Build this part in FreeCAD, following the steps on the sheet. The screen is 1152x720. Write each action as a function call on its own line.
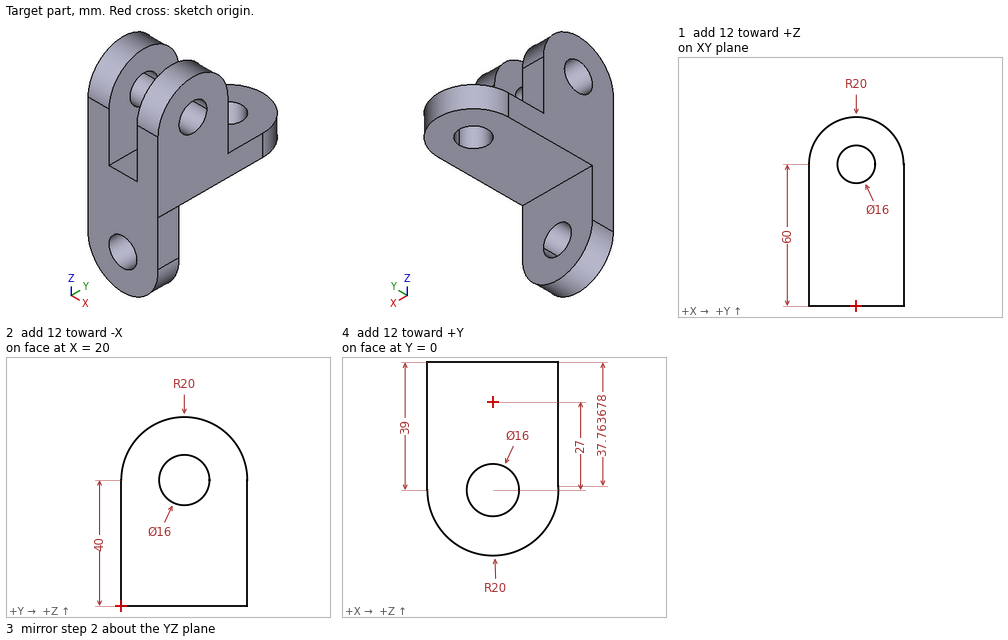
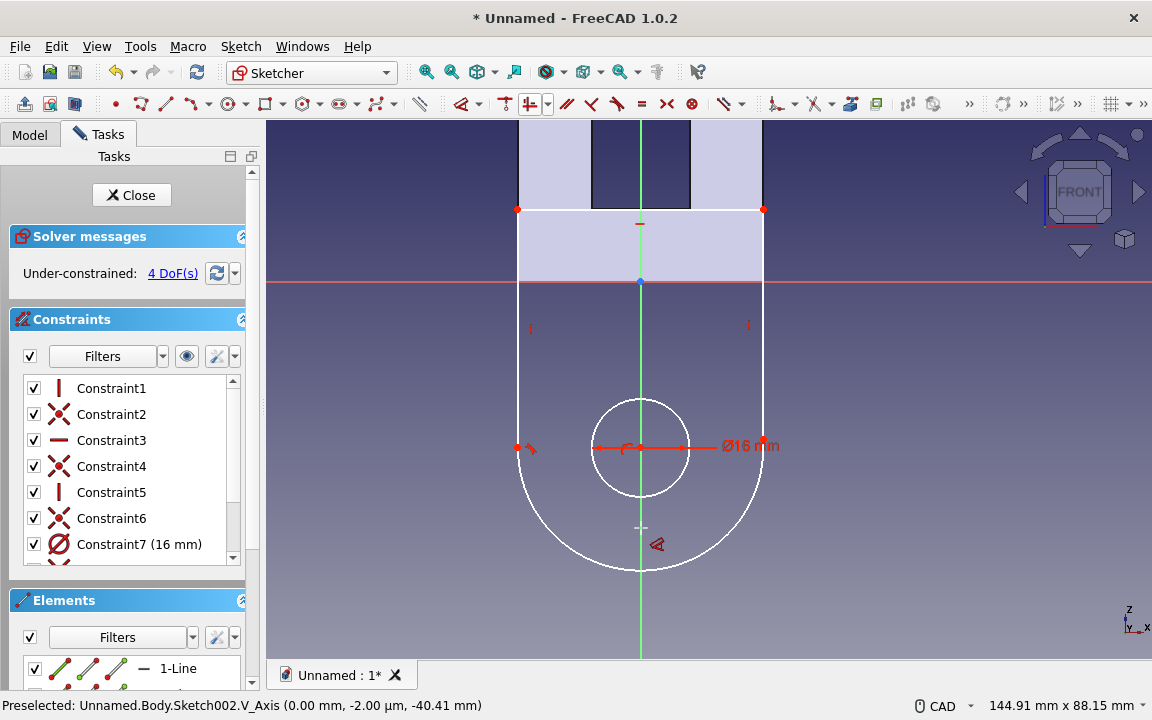
click(570, 549)
click(552, 575)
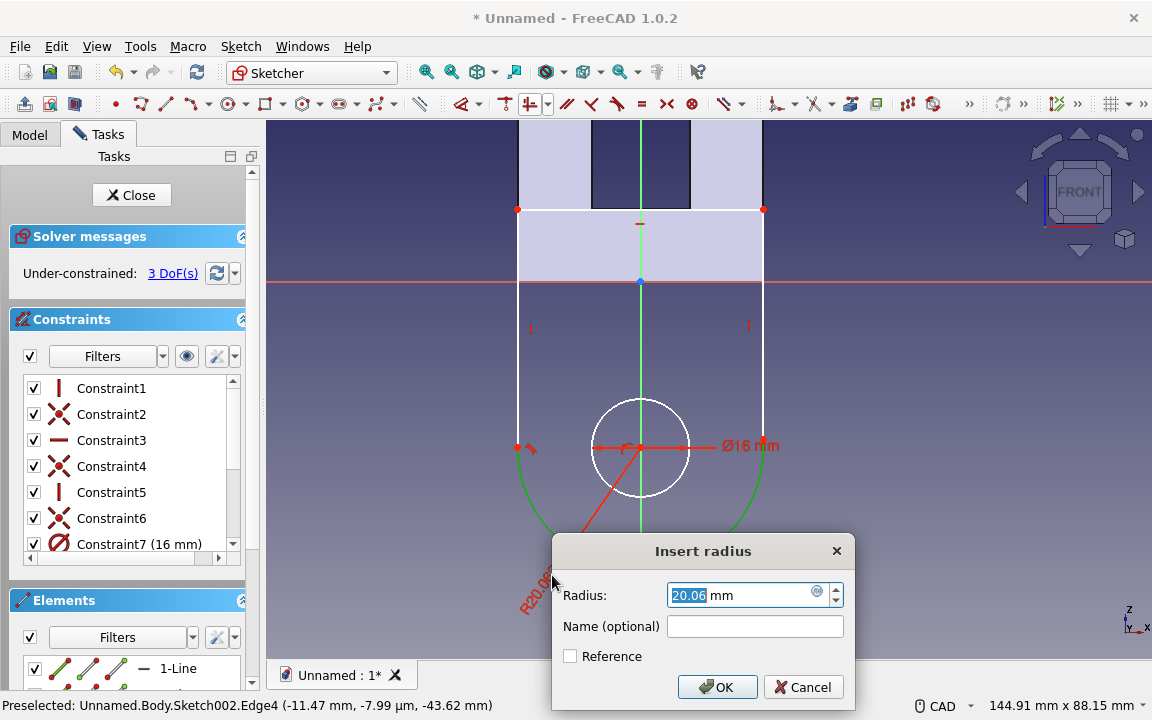
text(20)
key(Return)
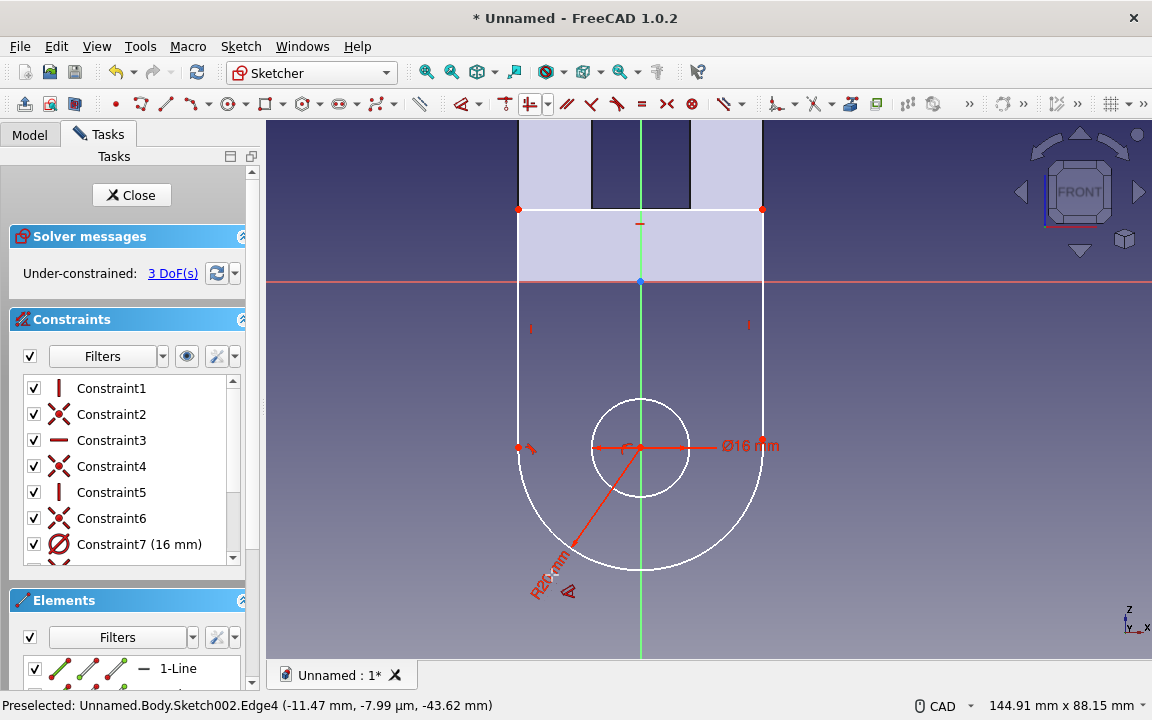
click(518, 281)
click(484, 329)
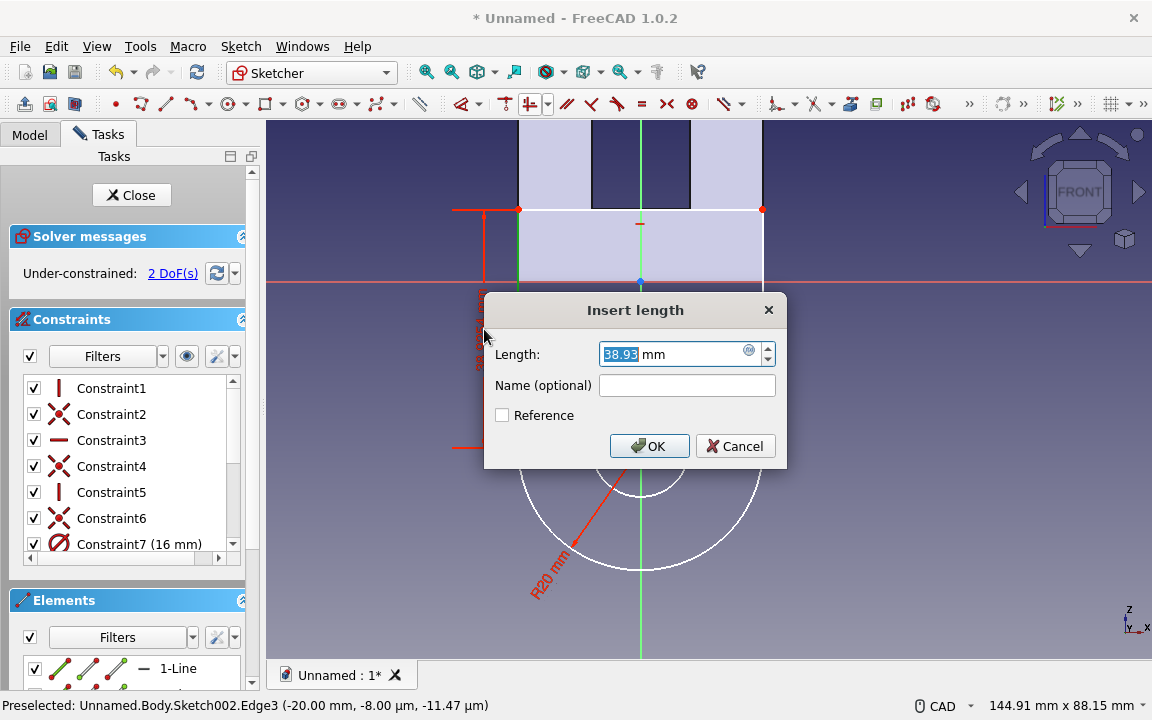
text(39)
key(Return)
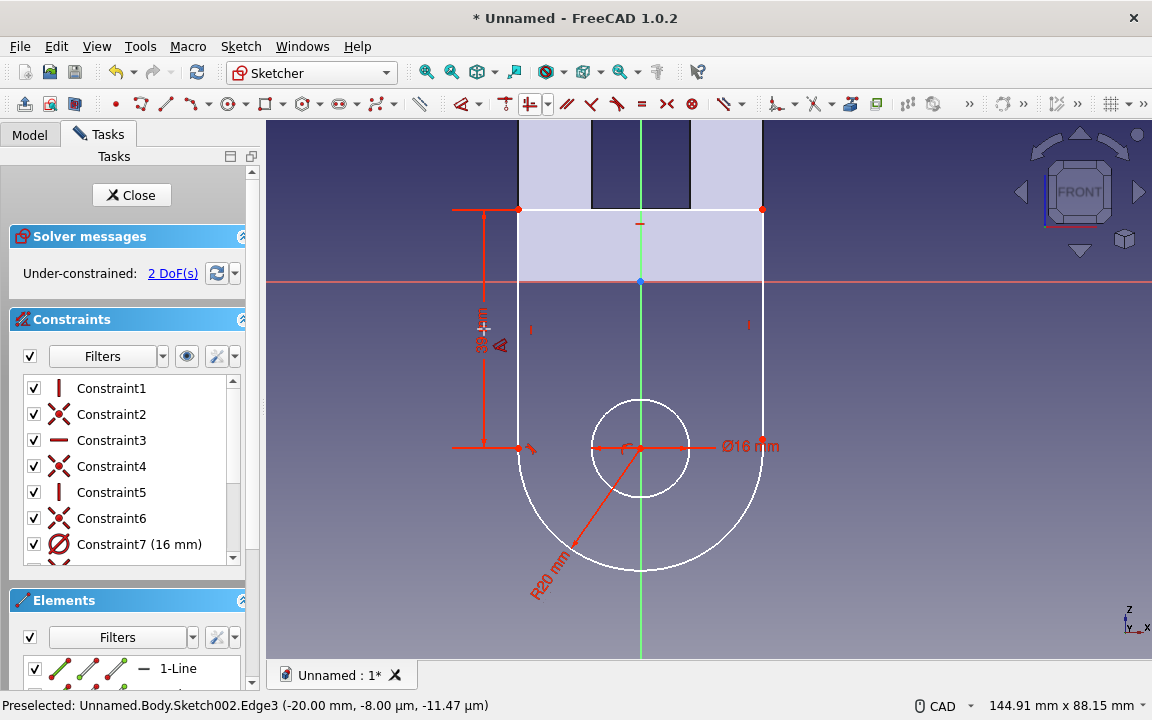
click(641, 448)
click(675, 365)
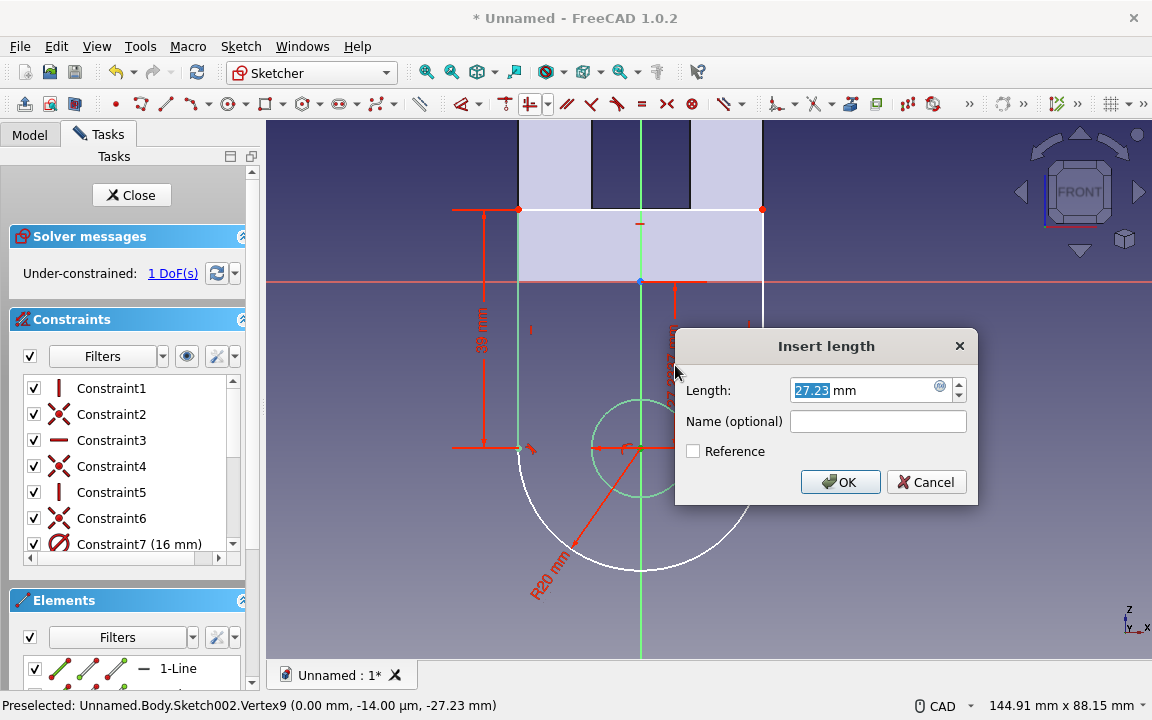
text(27)
key(Return)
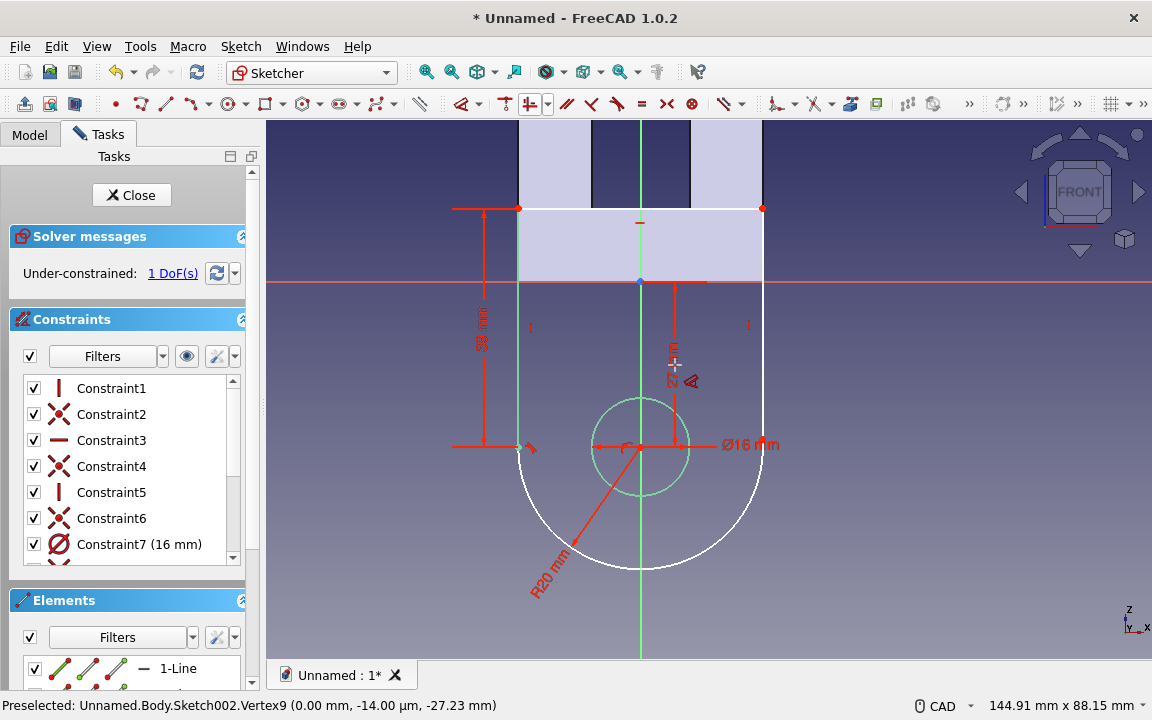
click(763, 371)
click(797, 324)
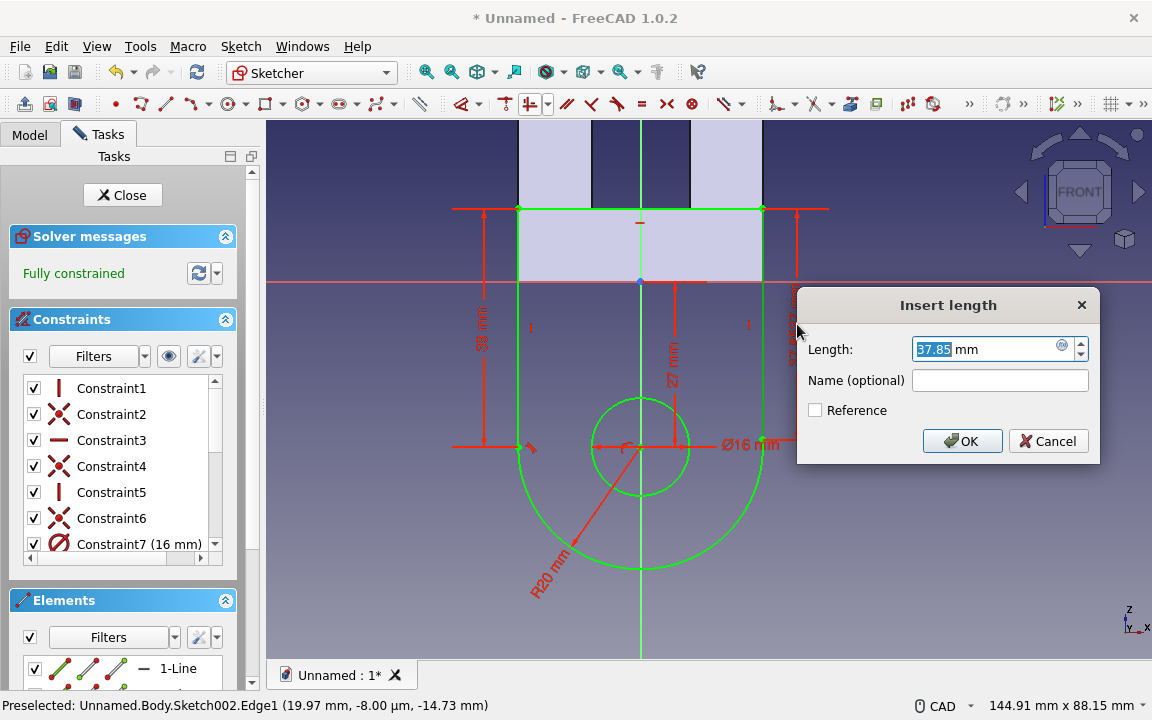
text(37.763678)
key(Return)
key(Escape)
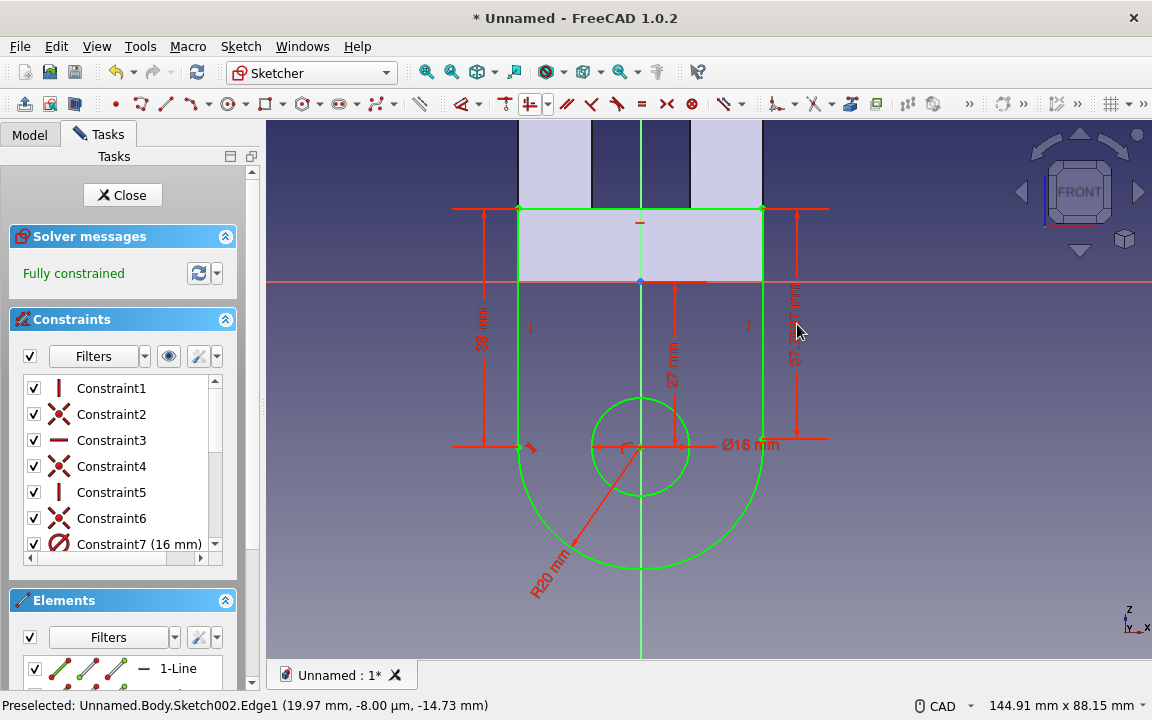
click(123, 195)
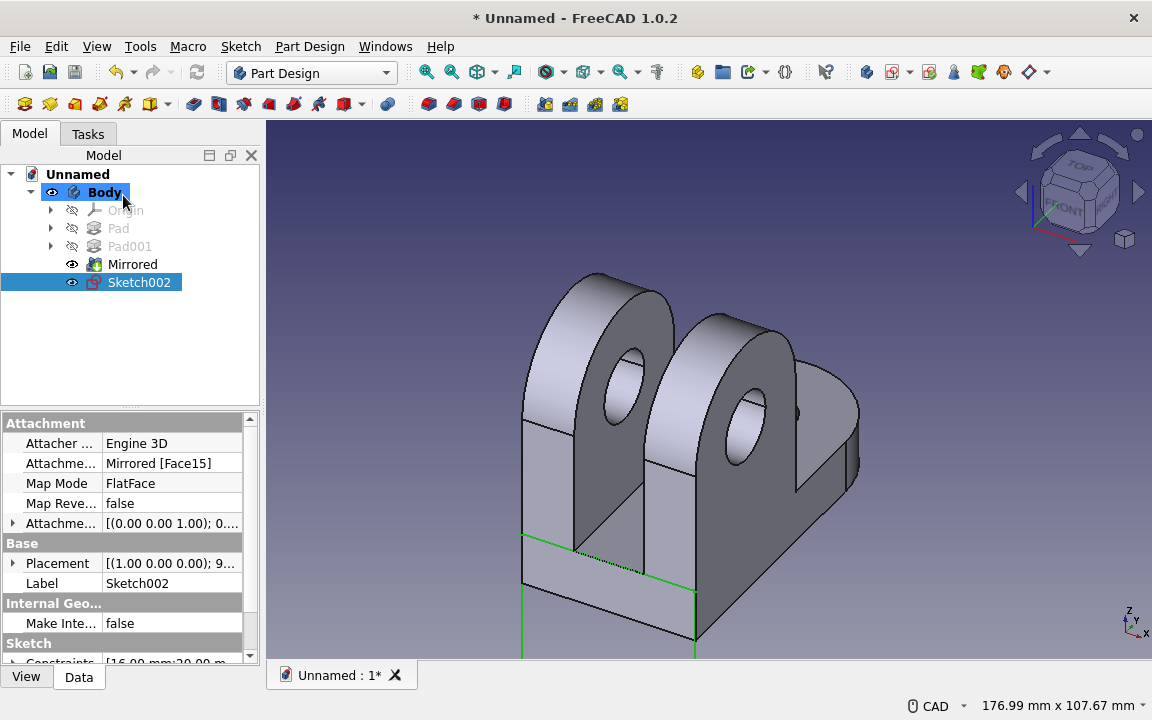
click(25, 104)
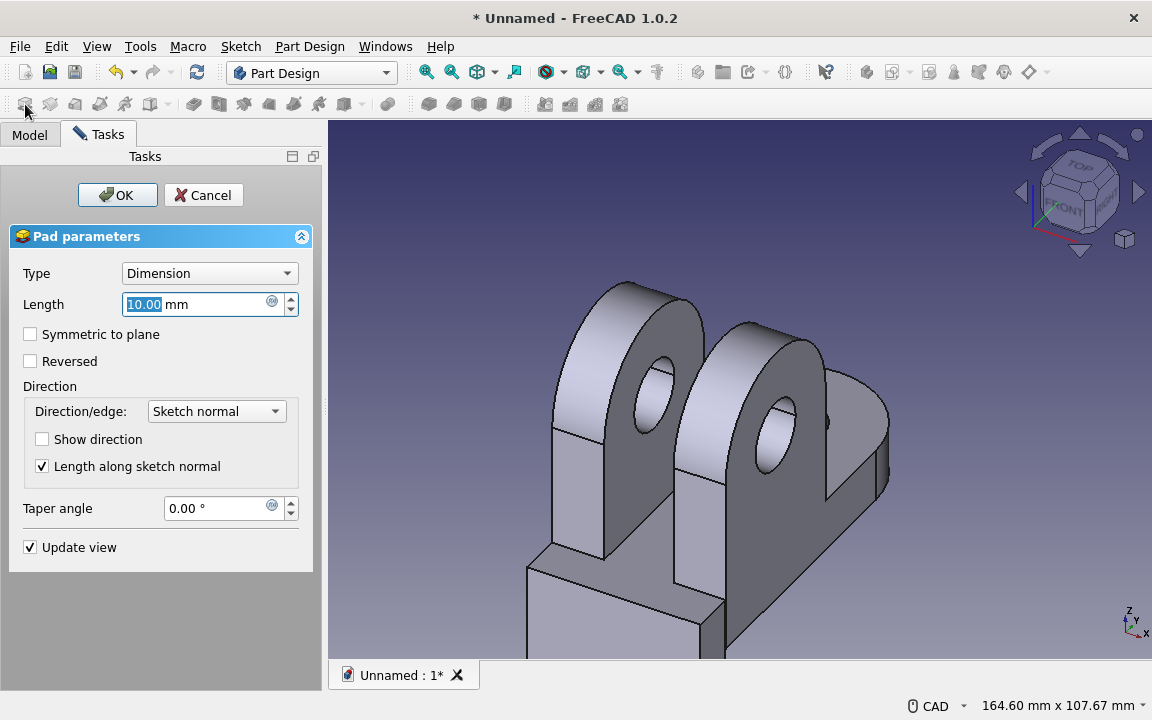
text(12)
key(Tab)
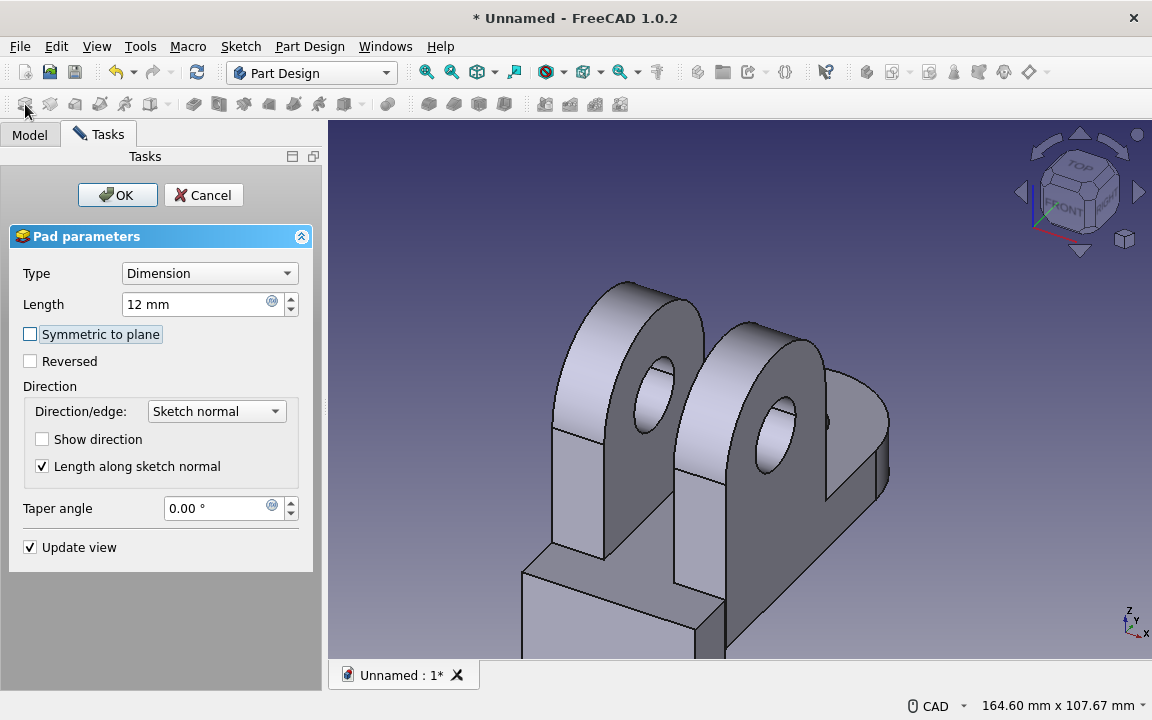
click(31, 361)